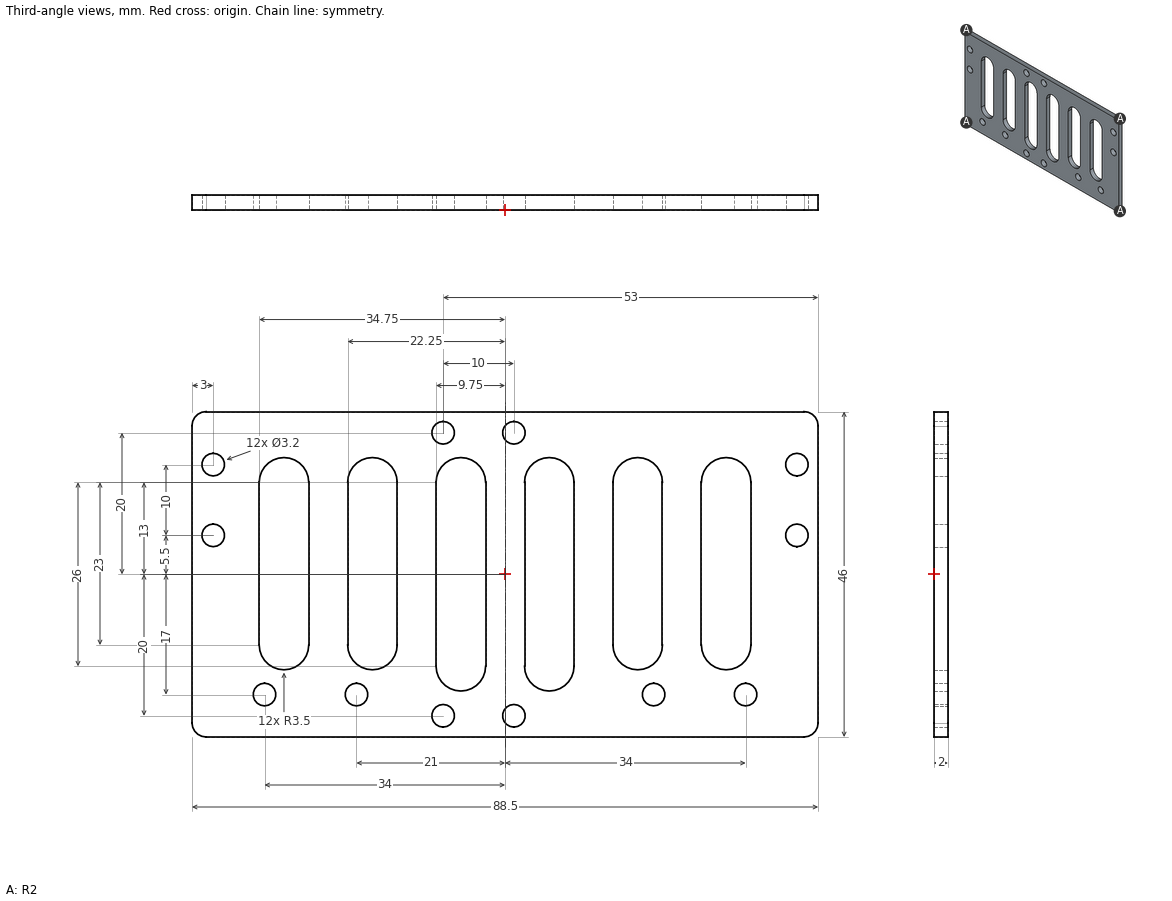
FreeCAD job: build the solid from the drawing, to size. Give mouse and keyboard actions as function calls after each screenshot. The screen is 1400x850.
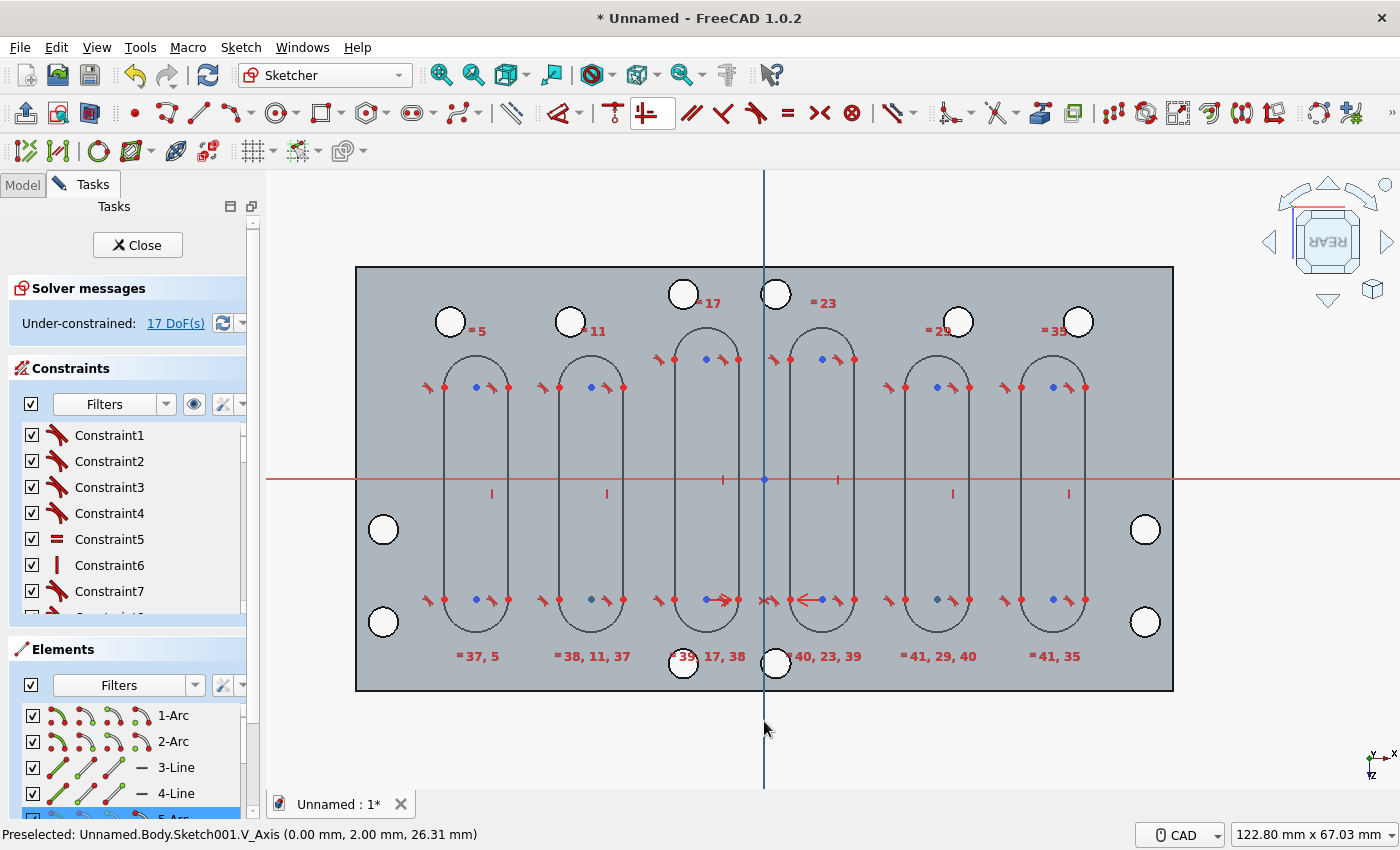
click(820, 114)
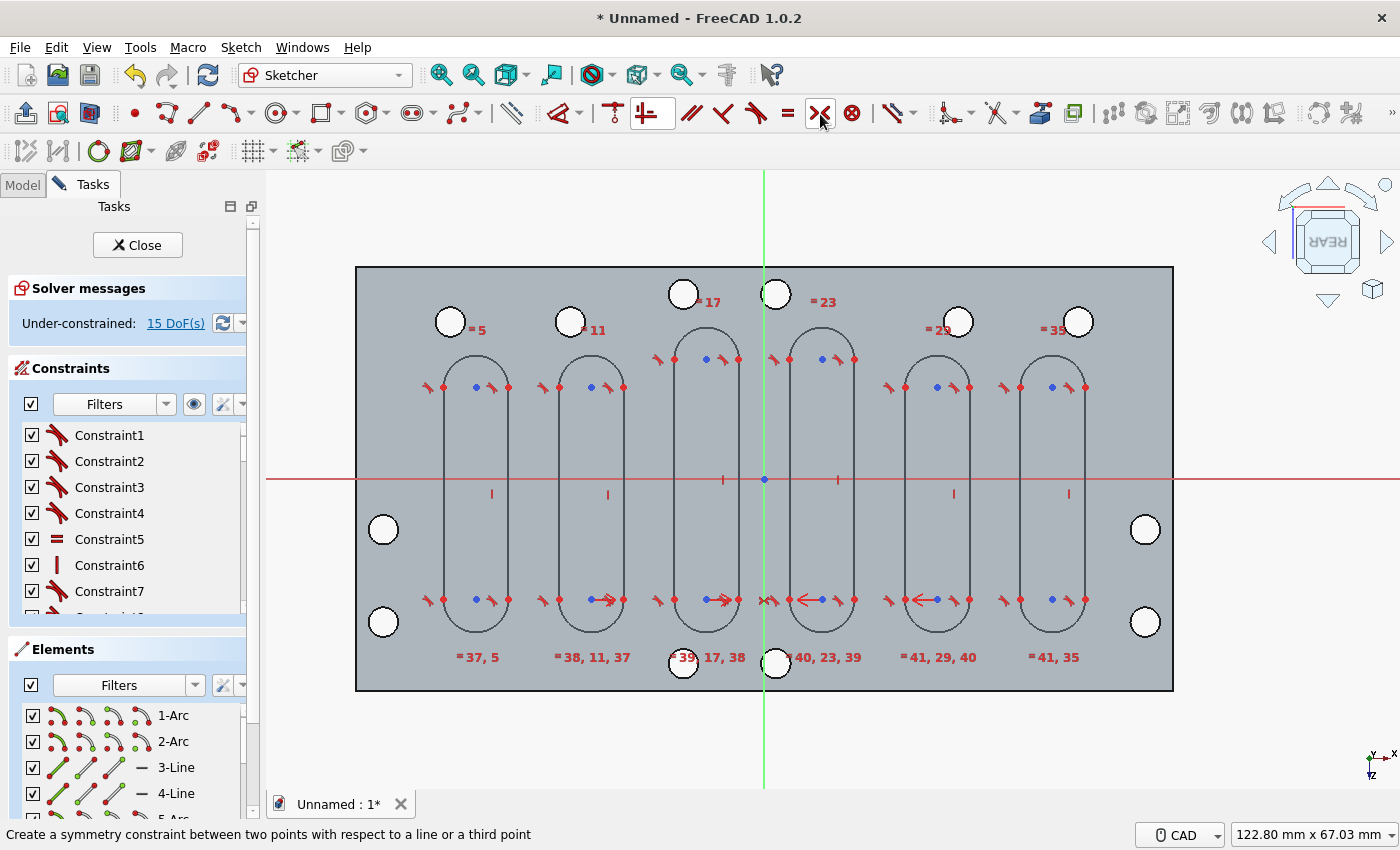
click(476, 600)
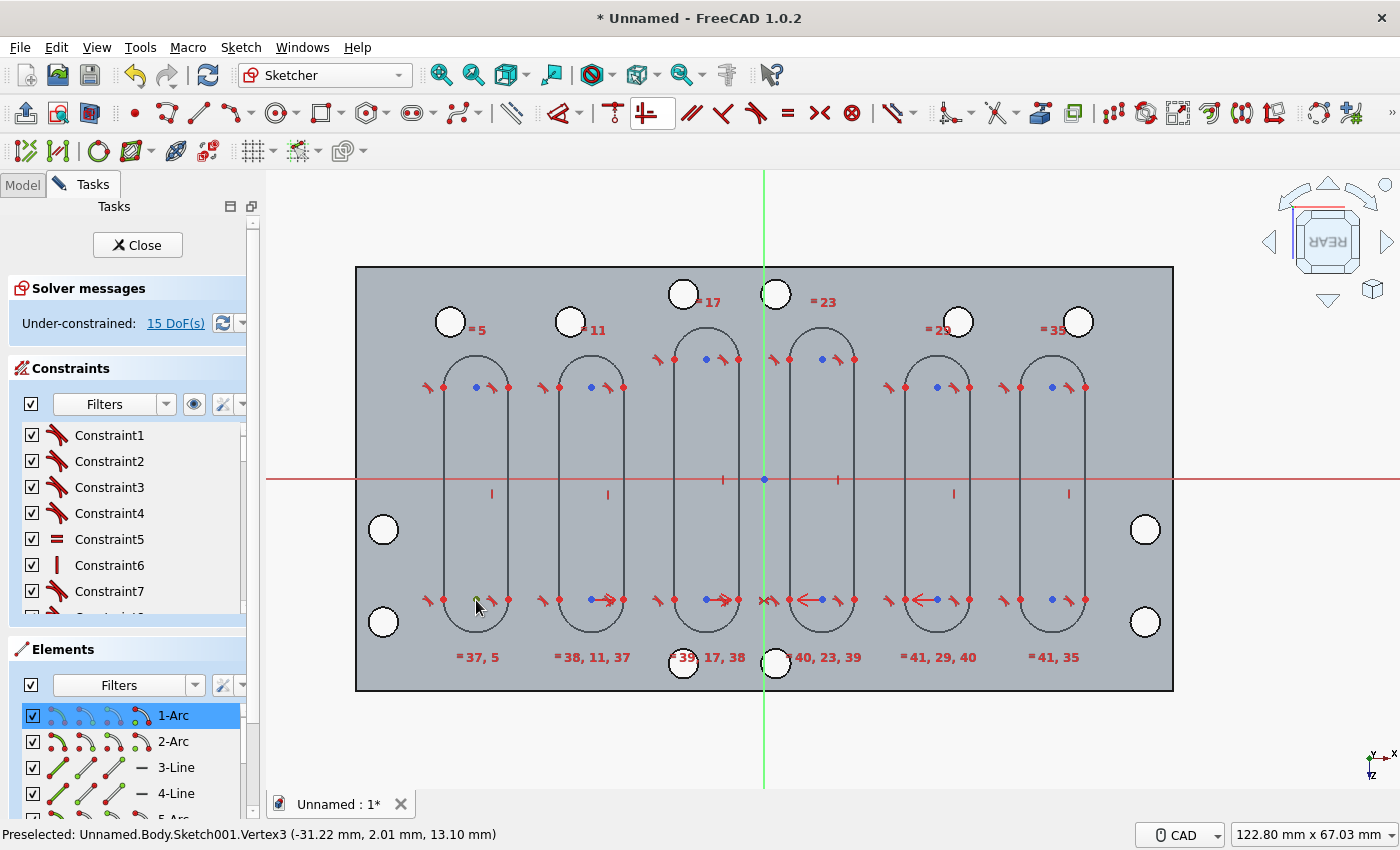
click(1053, 600)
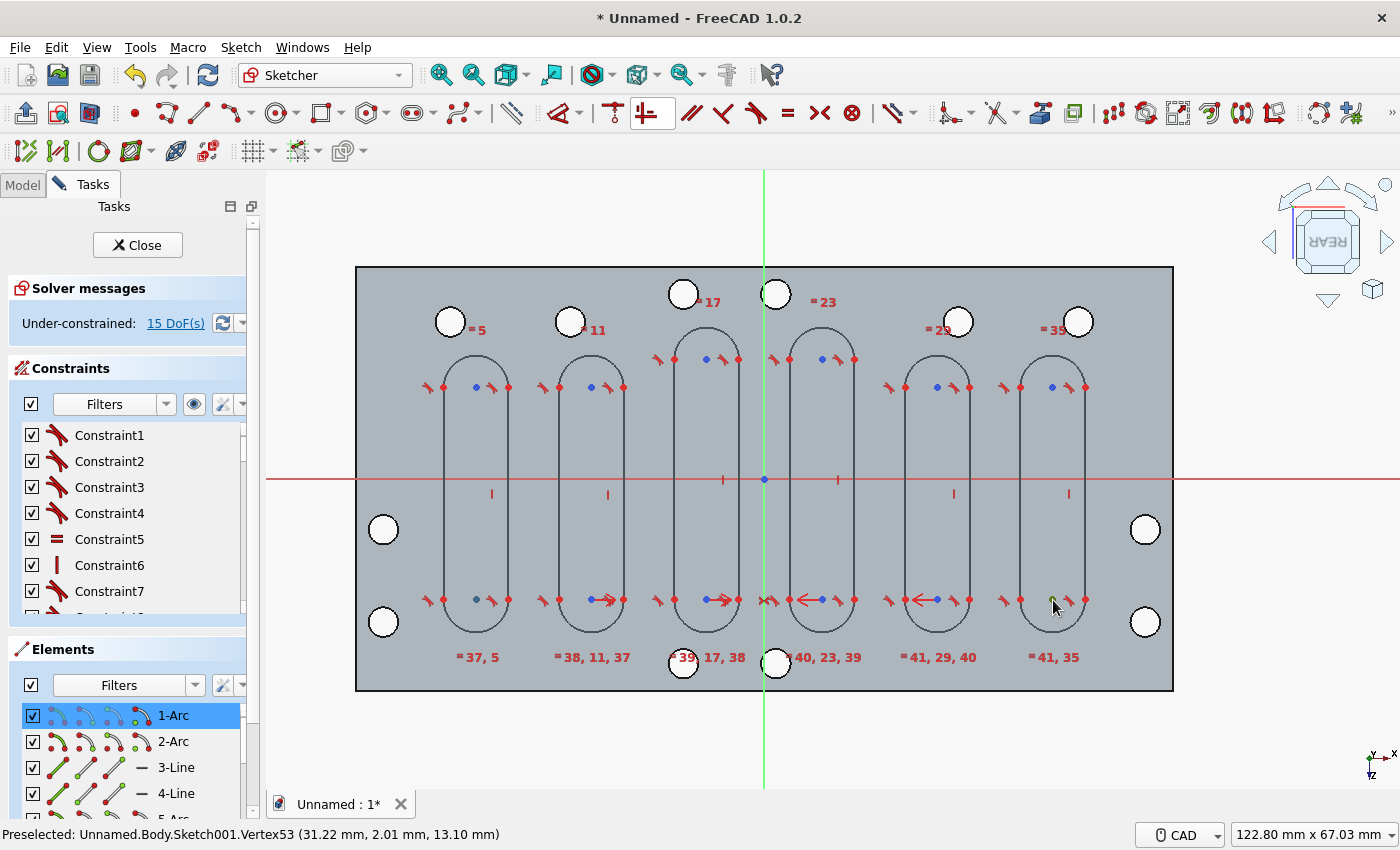
click(764, 721)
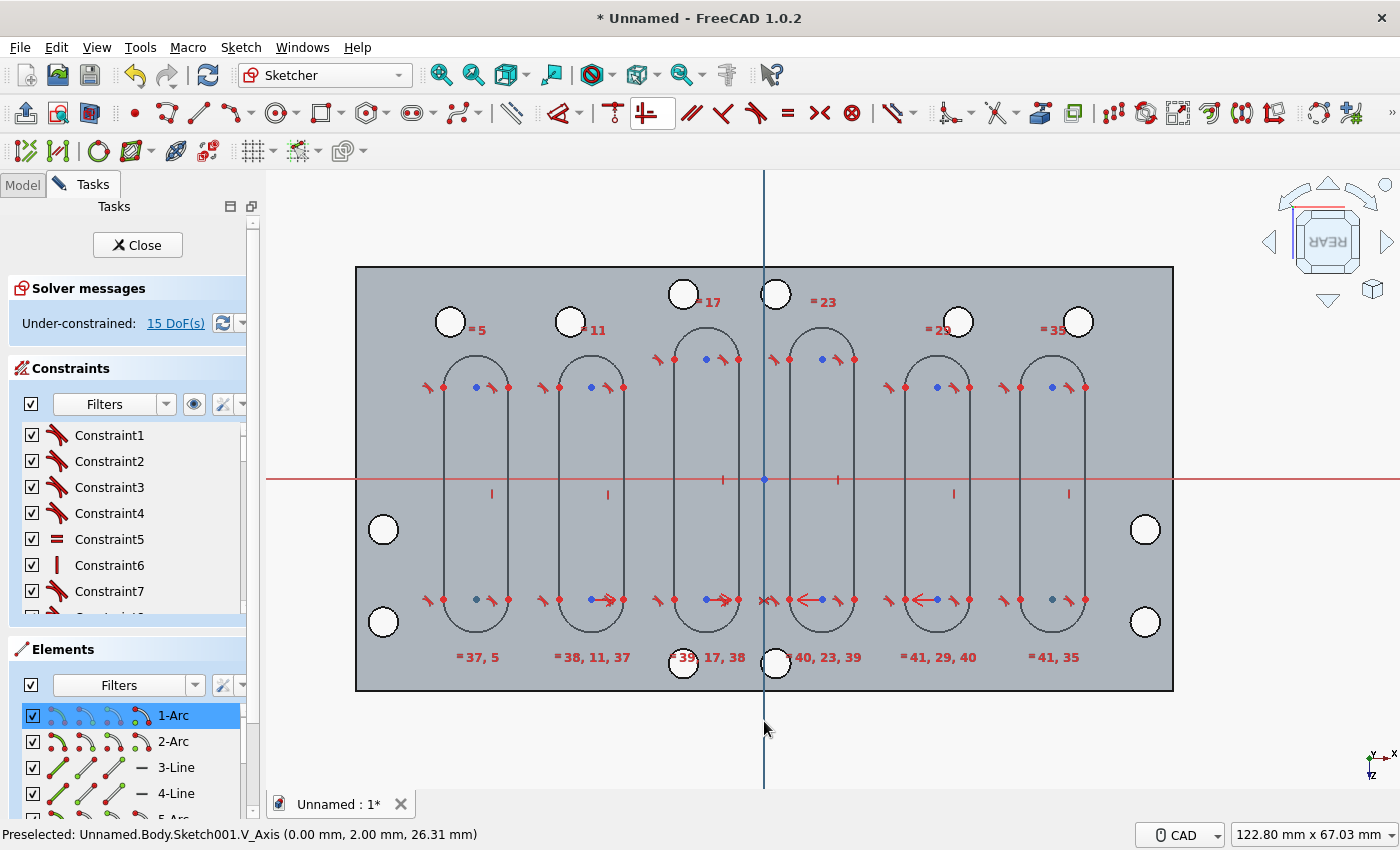
click(820, 114)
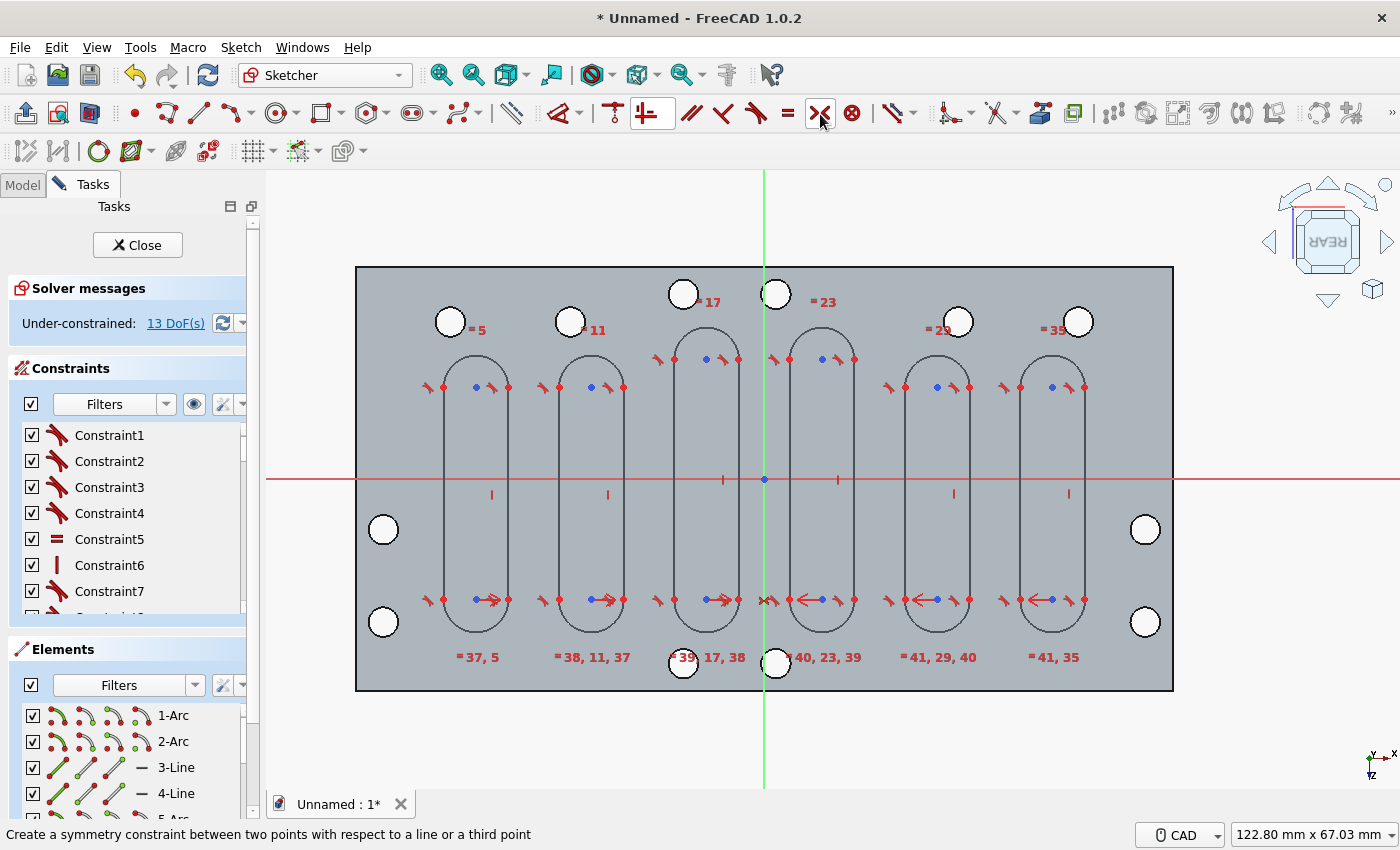
click(558, 114)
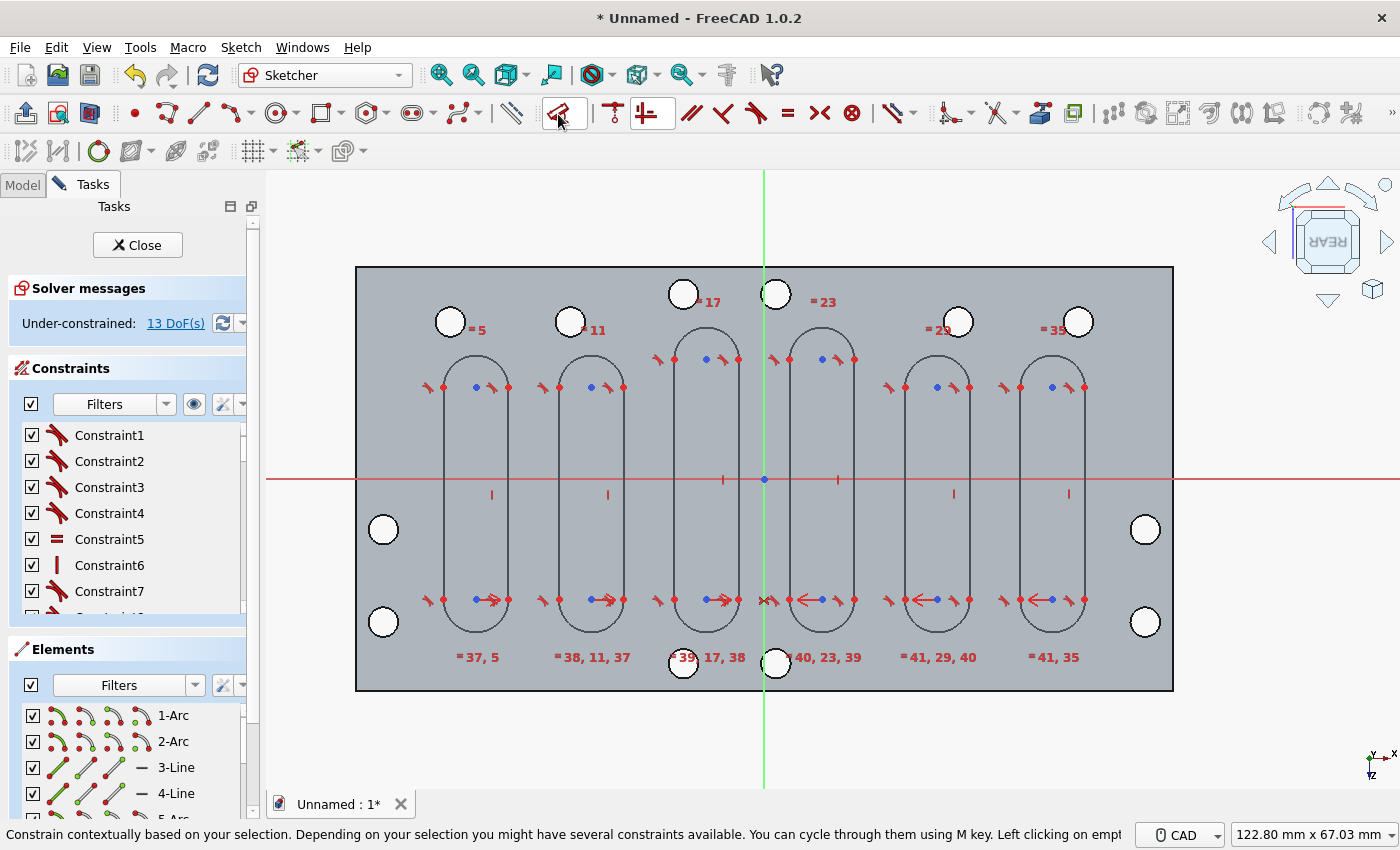
scroll(457, 626, up, 2)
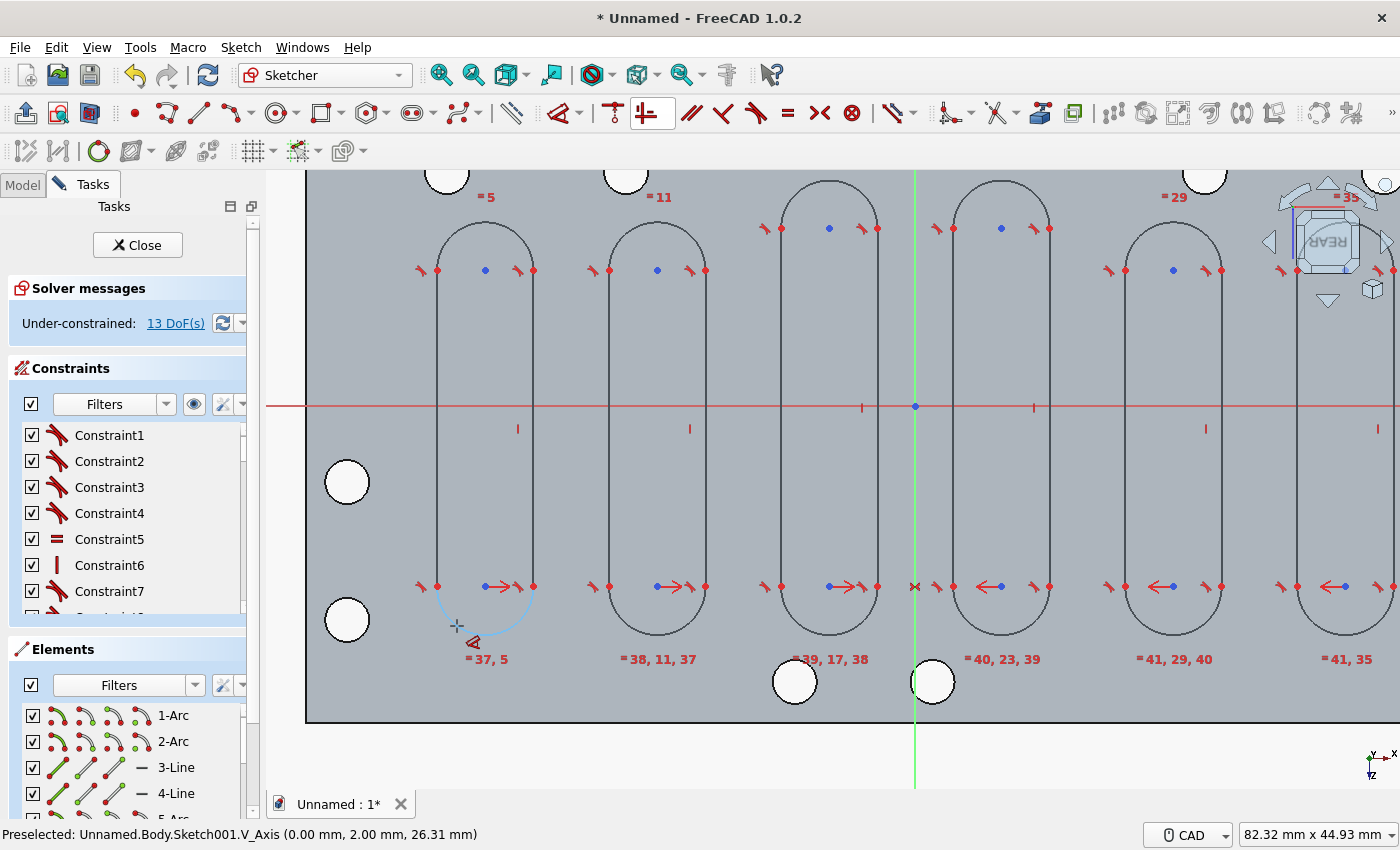
click(457, 626)
click(438, 652)